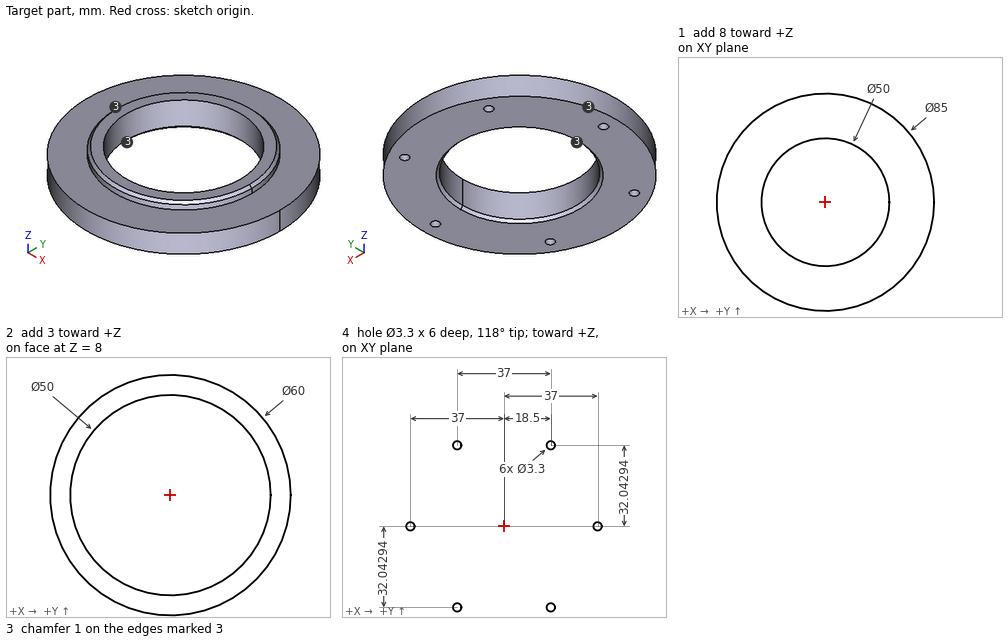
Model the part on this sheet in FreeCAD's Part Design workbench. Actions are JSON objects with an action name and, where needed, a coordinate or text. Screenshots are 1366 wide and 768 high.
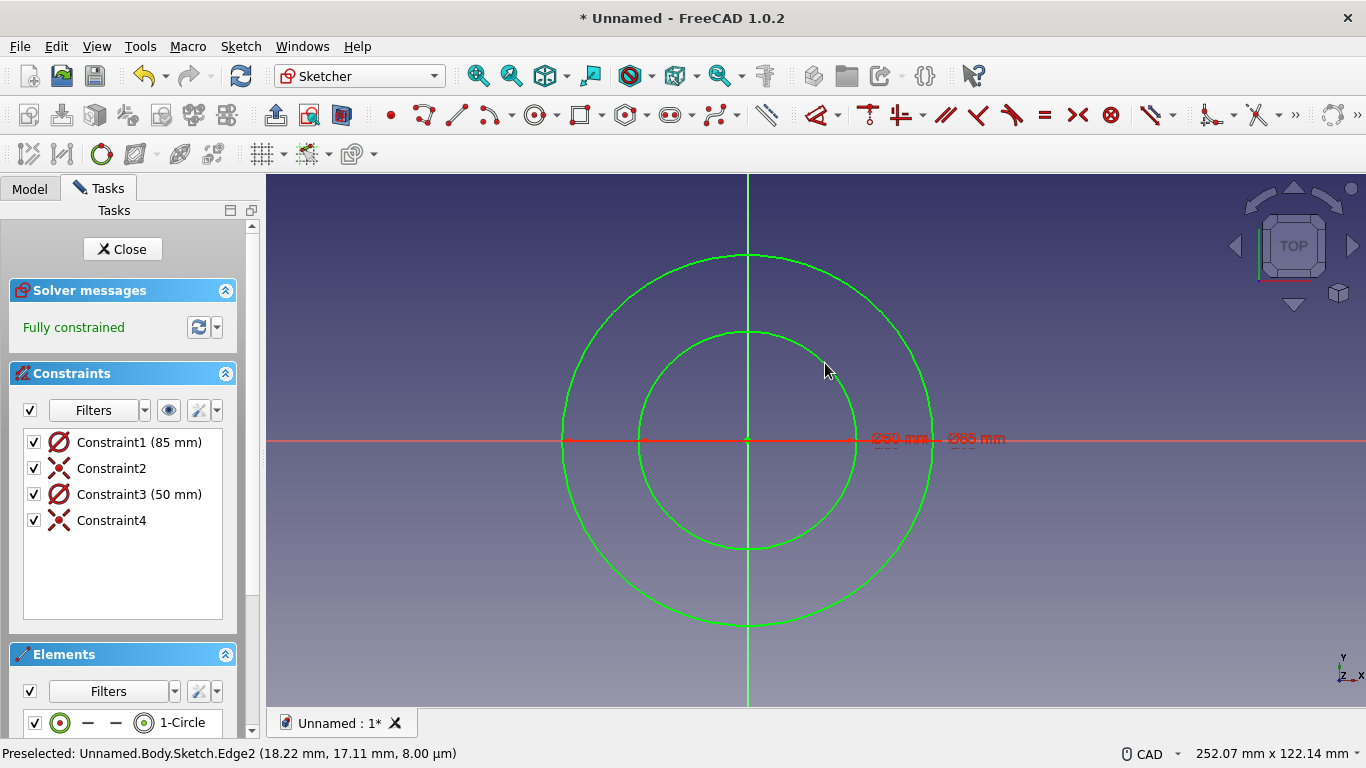
{"action": "left_click", "coordinate": [123, 249]}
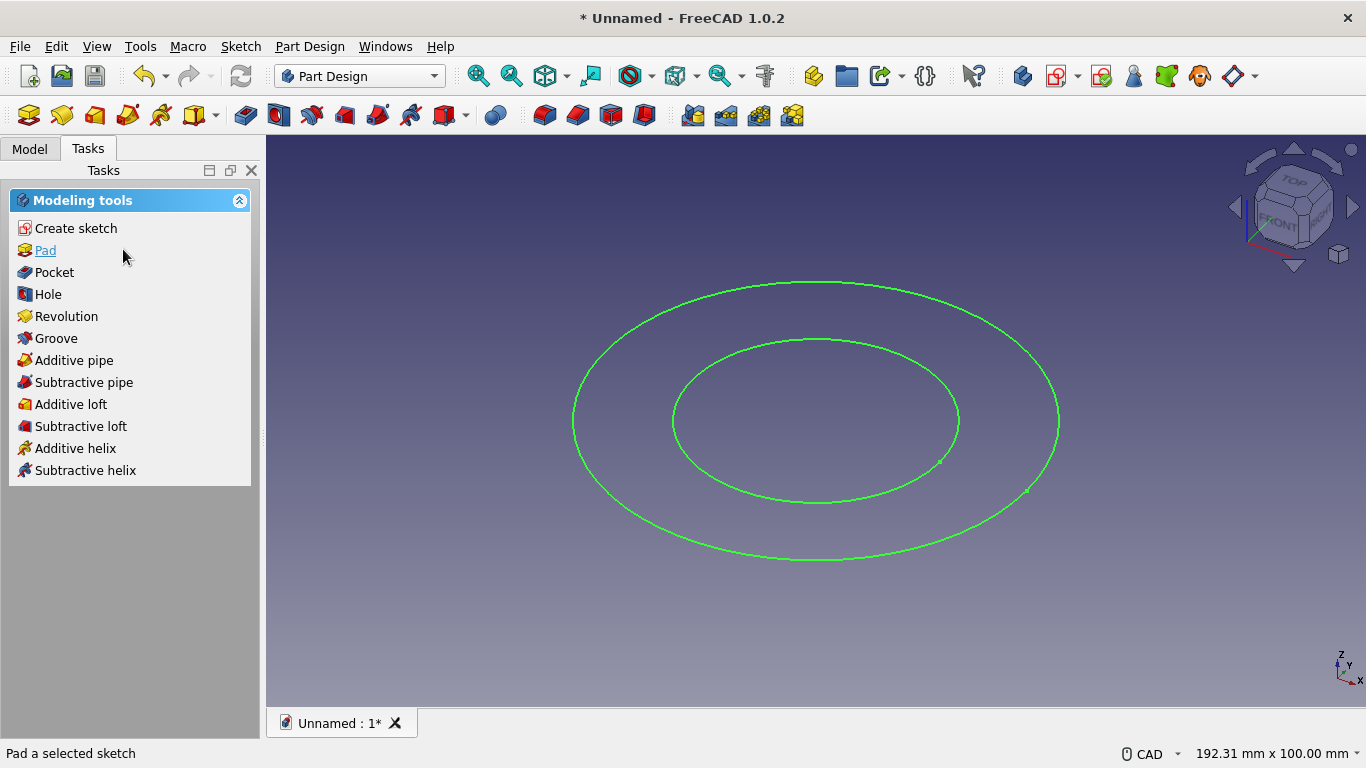
{"action": "left_click", "coordinate": [29, 116]}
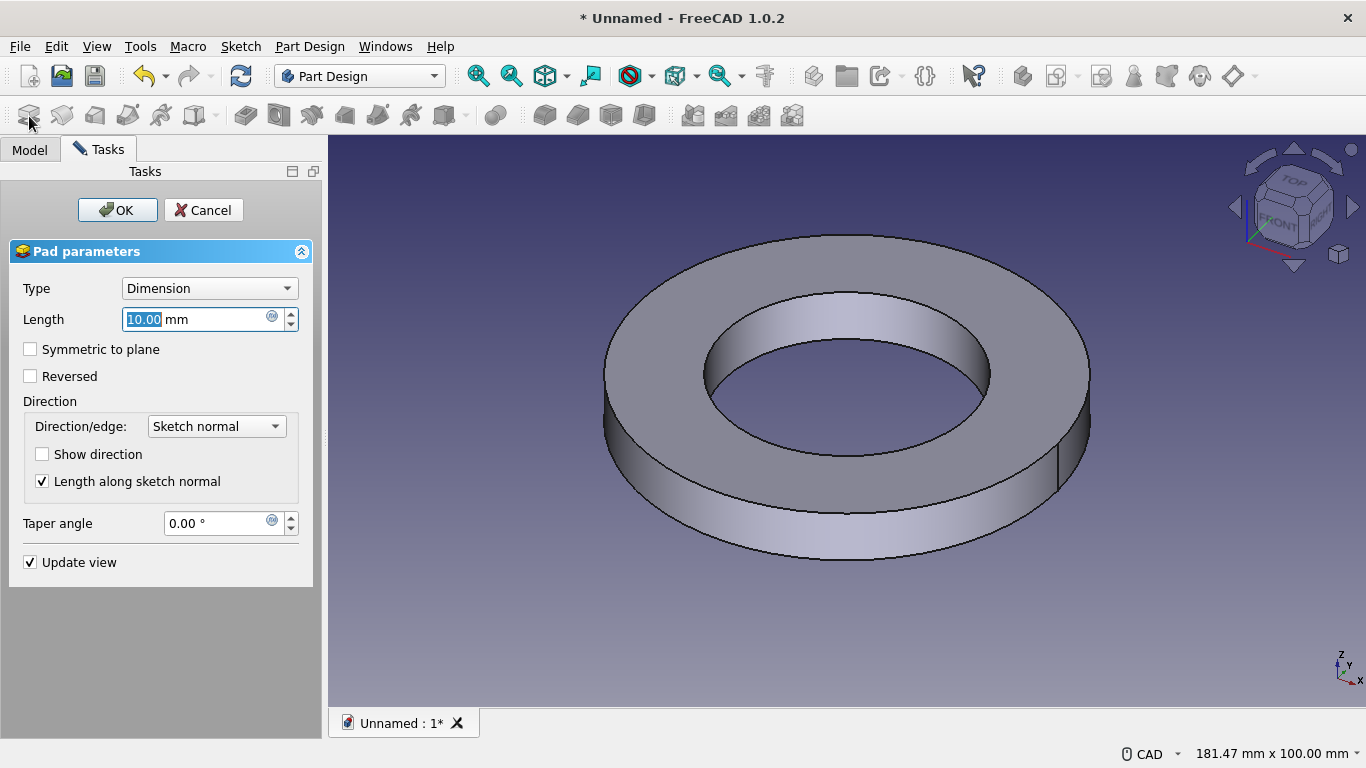
{"action": "type", "text": "8"}
{"action": "key", "text": "Tab"}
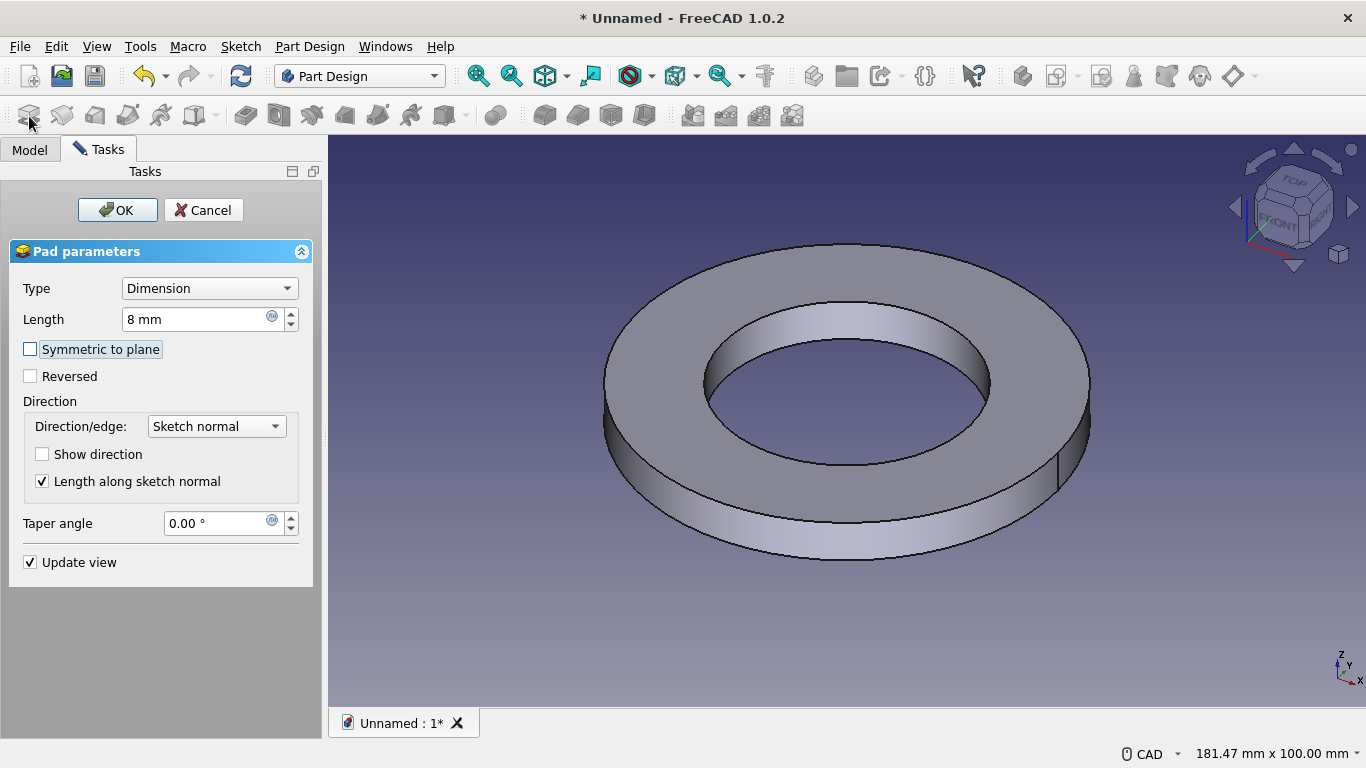
{"action": "left_click", "coordinate": [118, 210]}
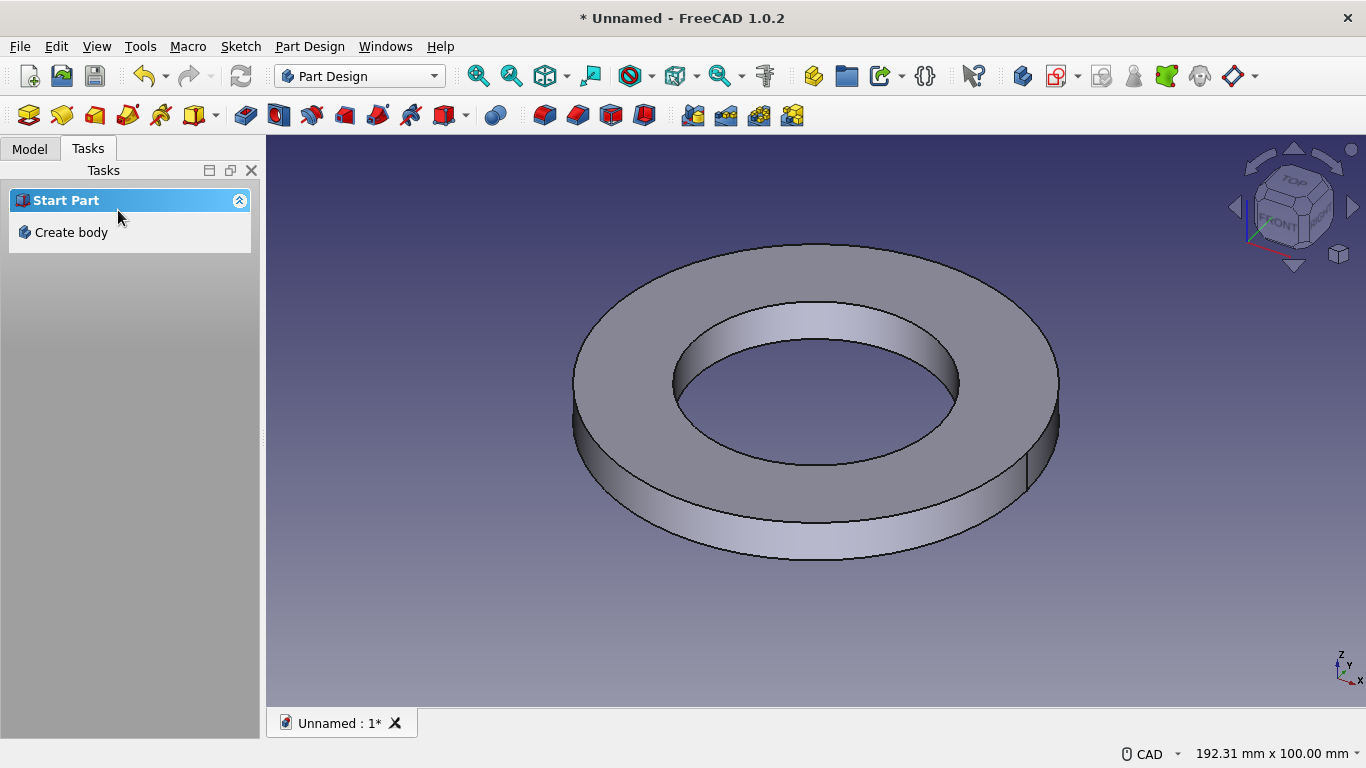
{"action": "left_click", "coordinate": [626, 412]}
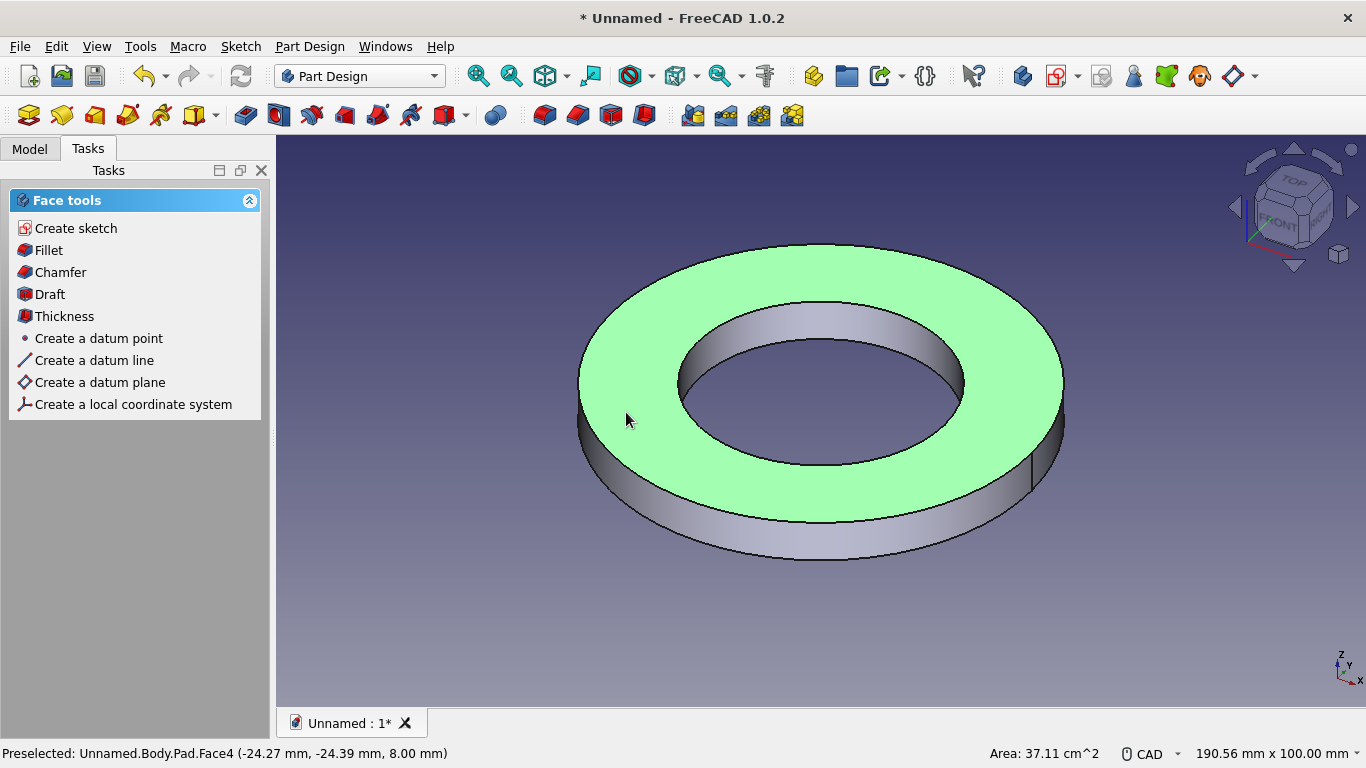
{"action": "left_click", "coordinate": [1056, 76]}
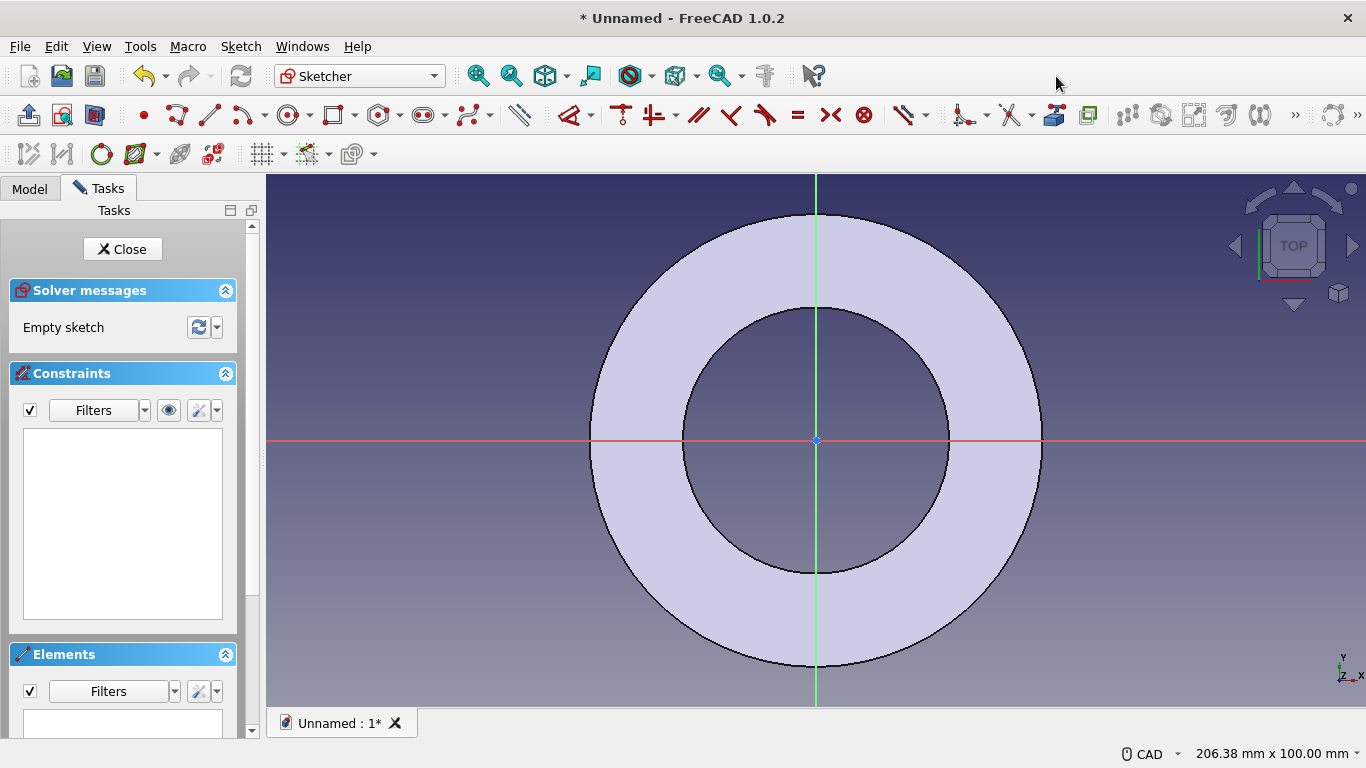
{"action": "left_click", "coordinate": [288, 116]}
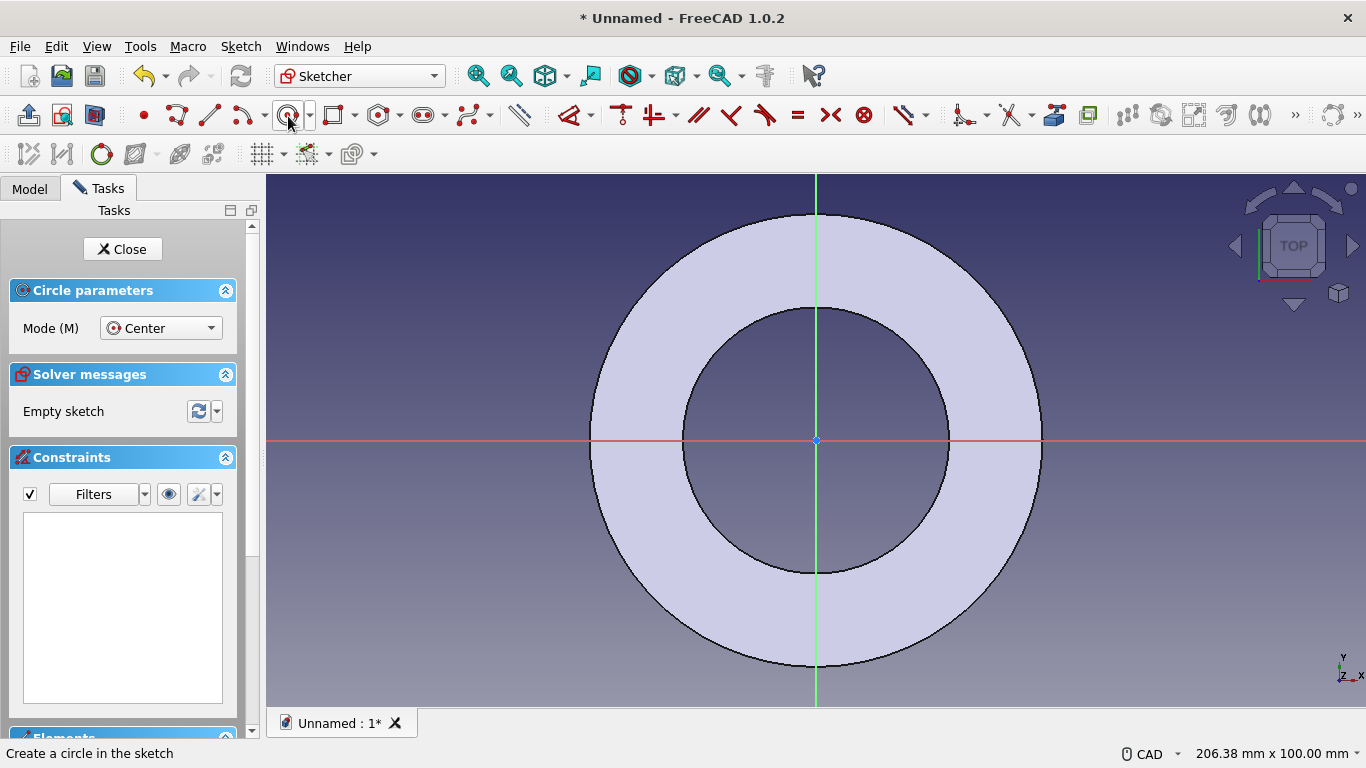
{"action": "left_click", "coordinate": [816, 440]}
{"action": "mouse_move", "coordinate": [929, 327]}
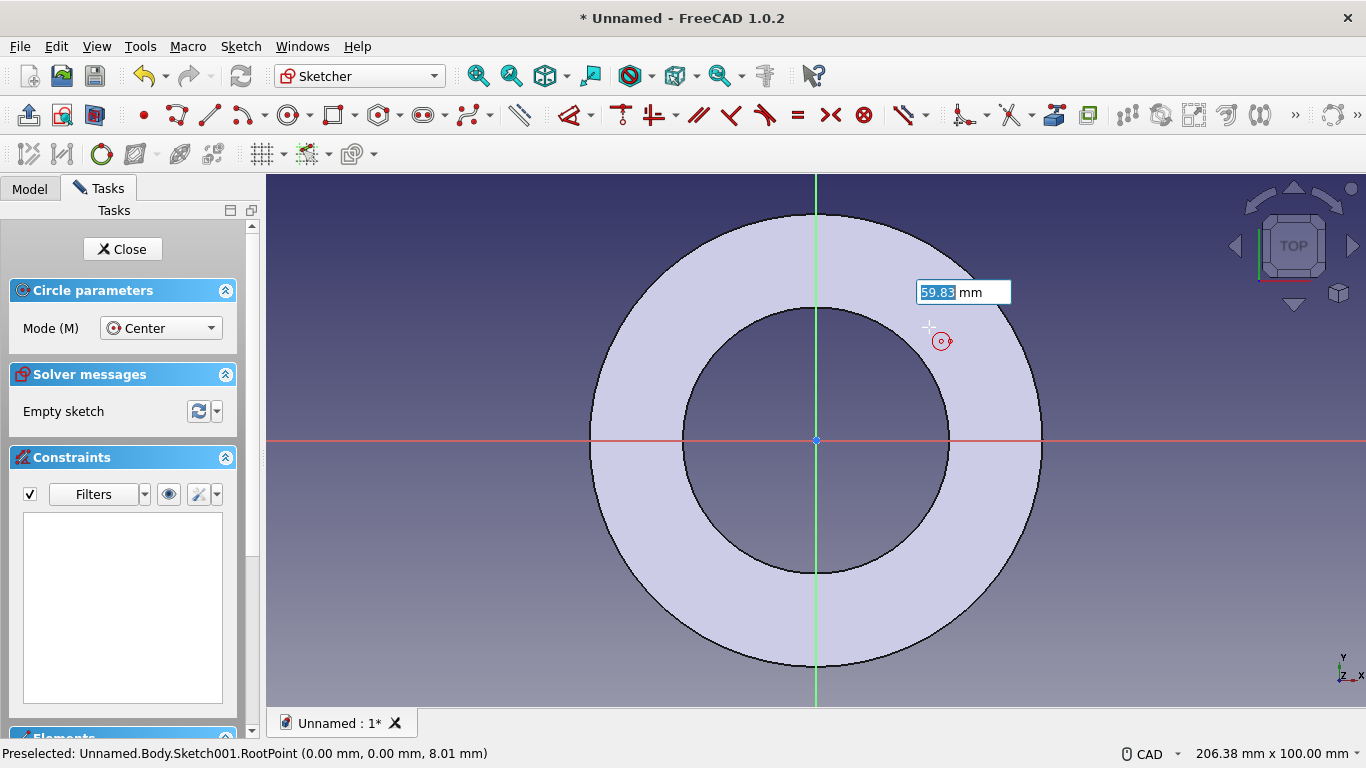
{"action": "type", "text": "60"}
{"action": "key", "text": "Return"}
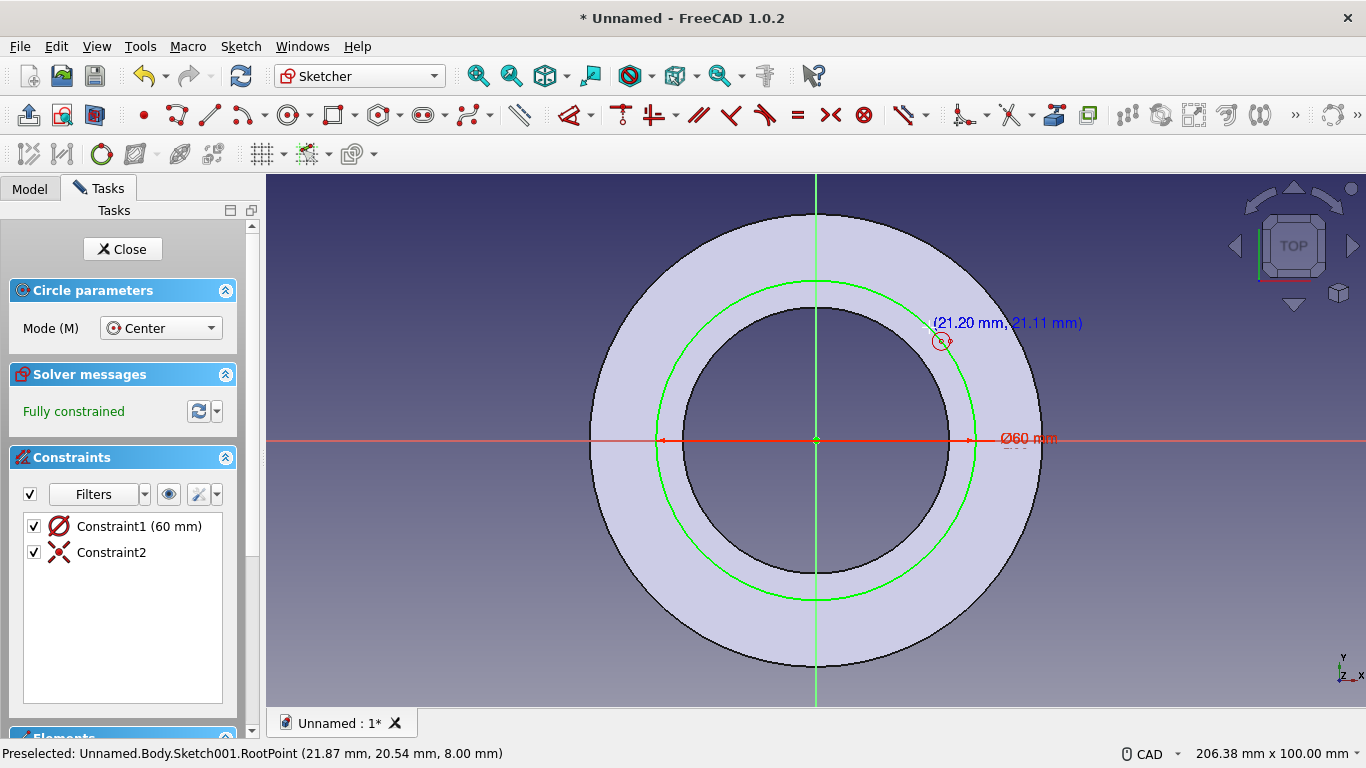
{"action": "left_click", "coordinate": [816, 440]}
{"action": "mouse_move", "coordinate": [910, 346]}